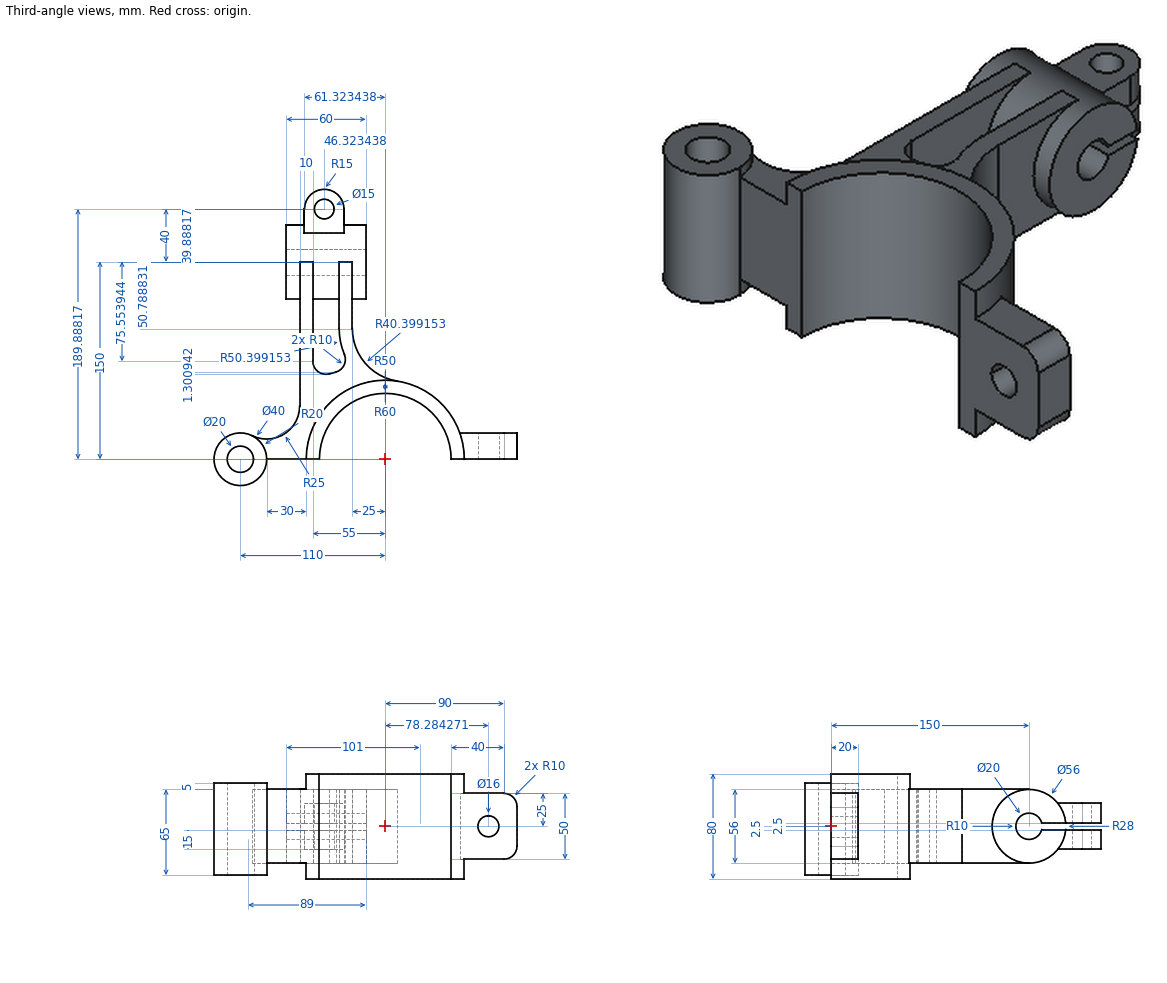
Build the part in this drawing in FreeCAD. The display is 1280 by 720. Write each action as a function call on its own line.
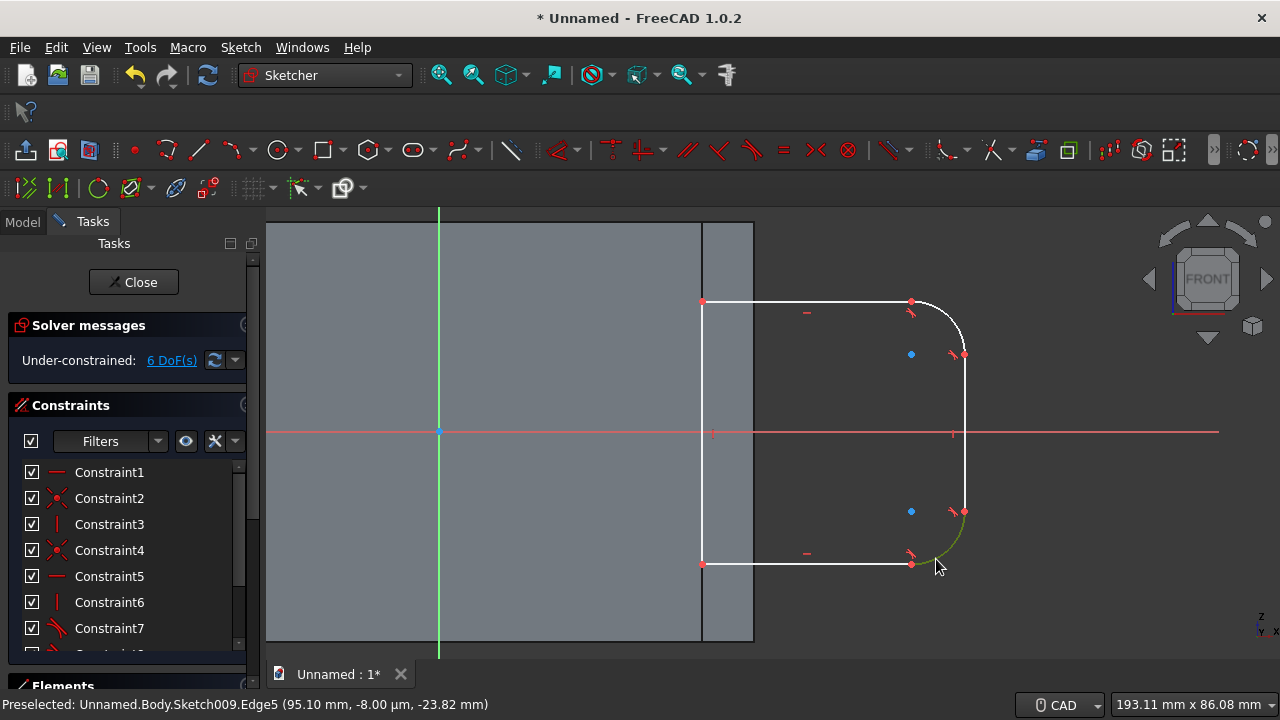
click(959, 330)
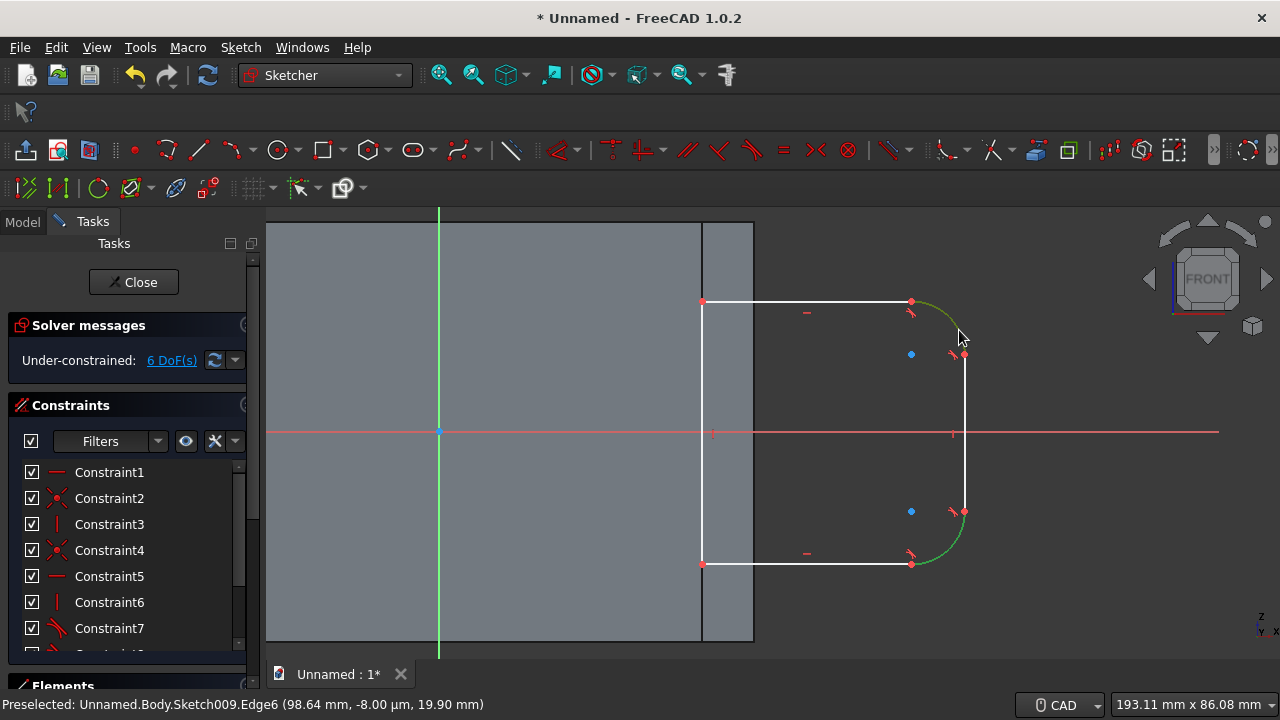
key(e)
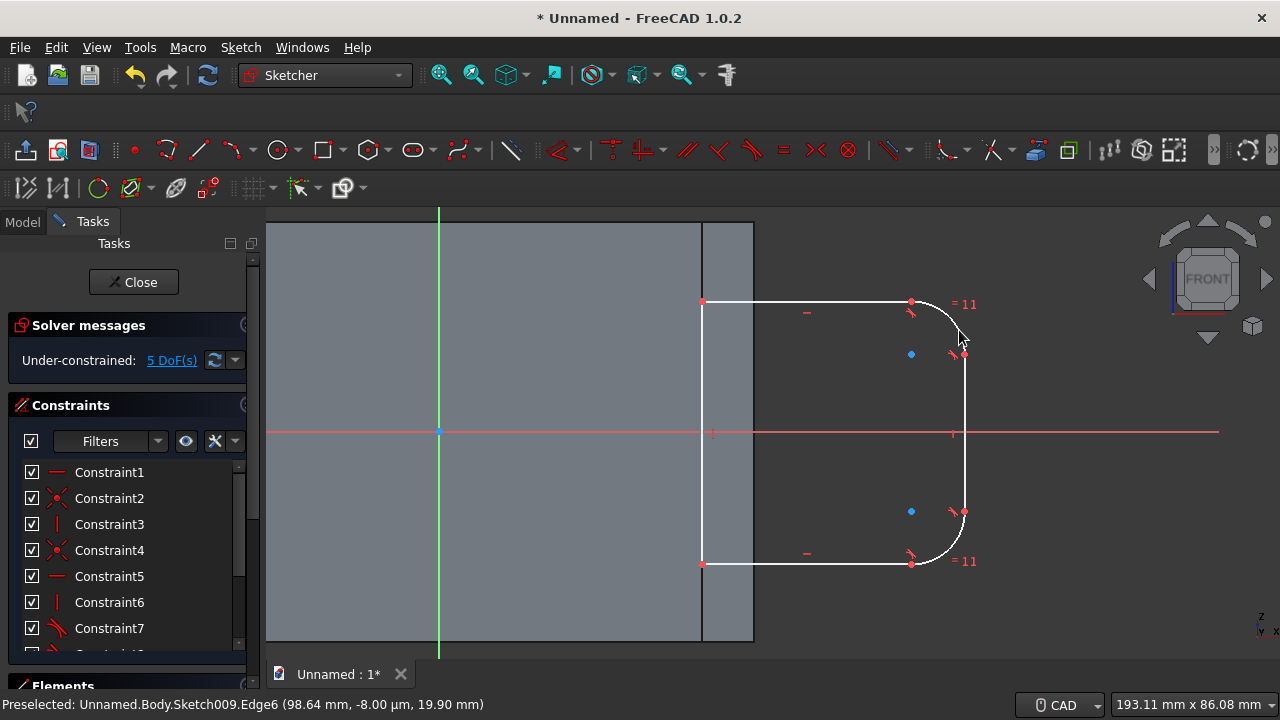
key(d)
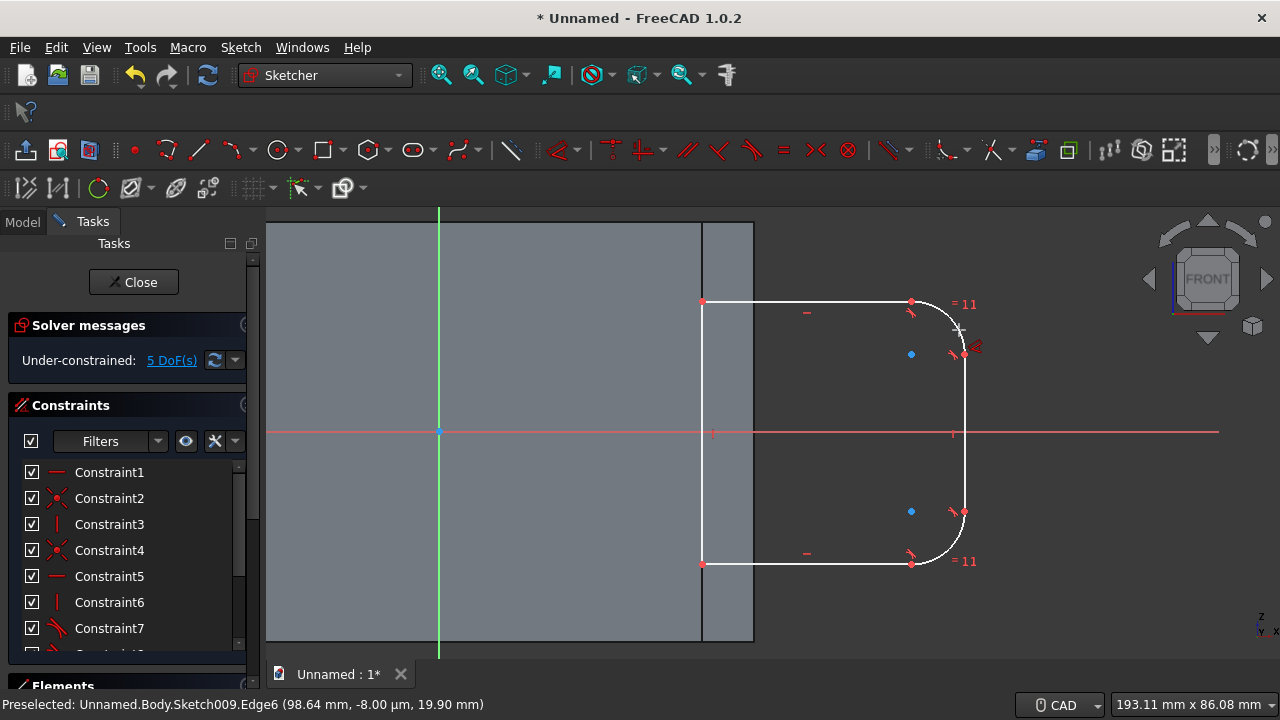
click(936, 559)
click(950, 588)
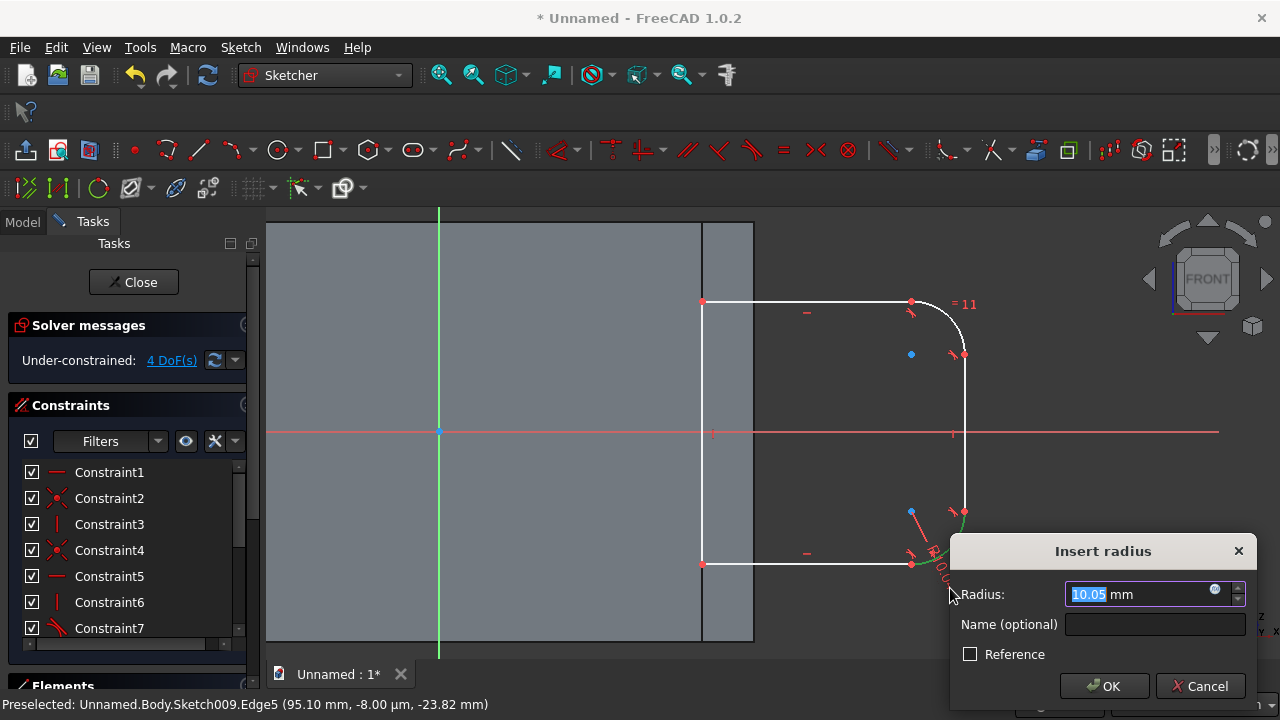
text(10)
key(Return)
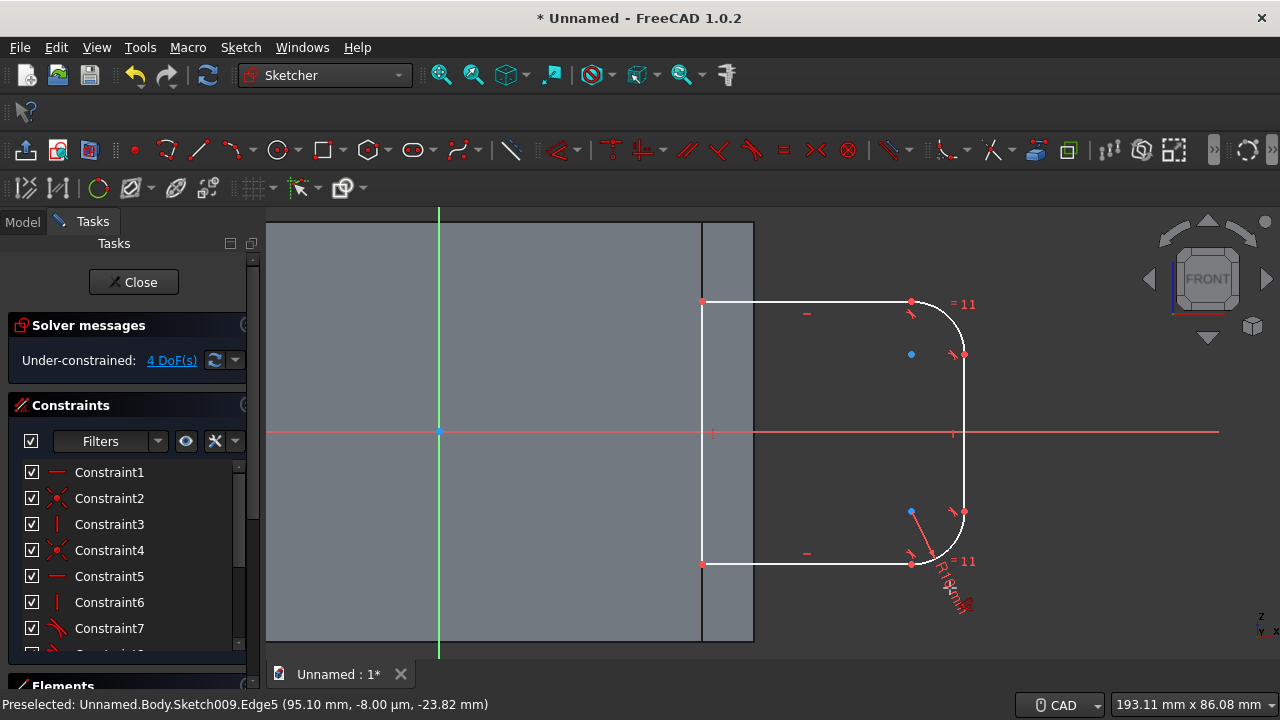
click(849, 302)
click(807, 268)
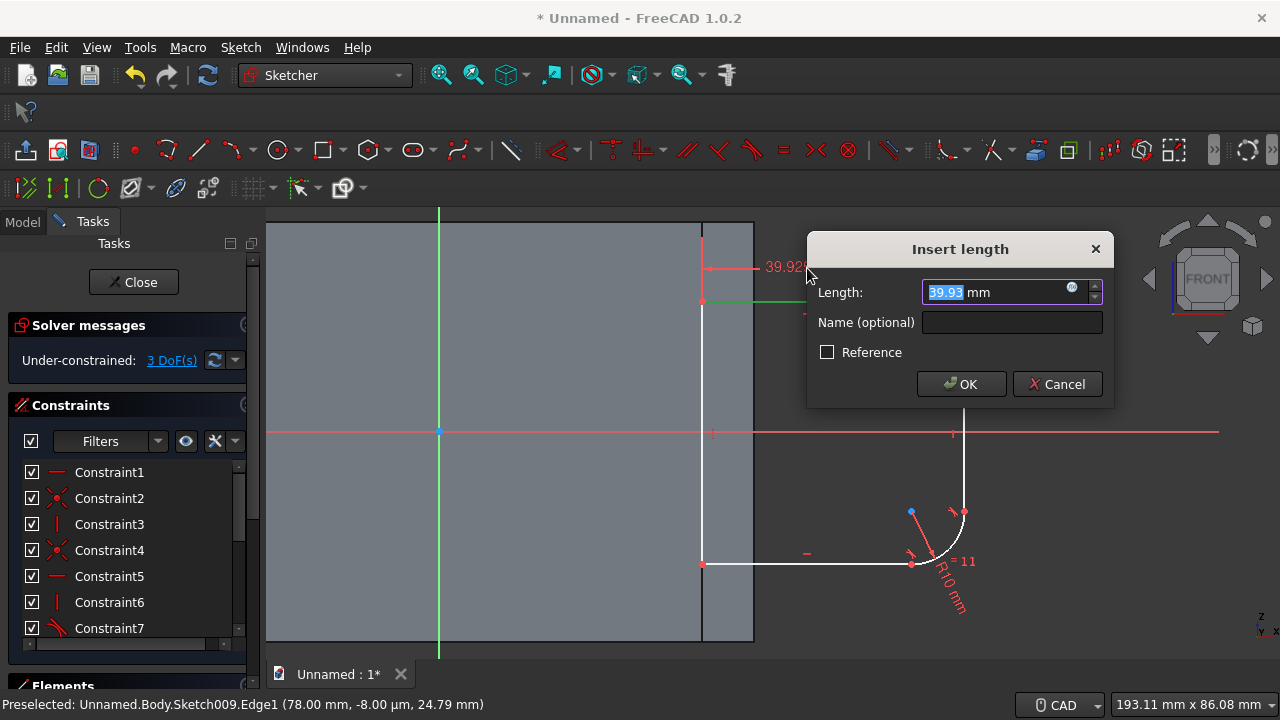
text(40)
key(Return)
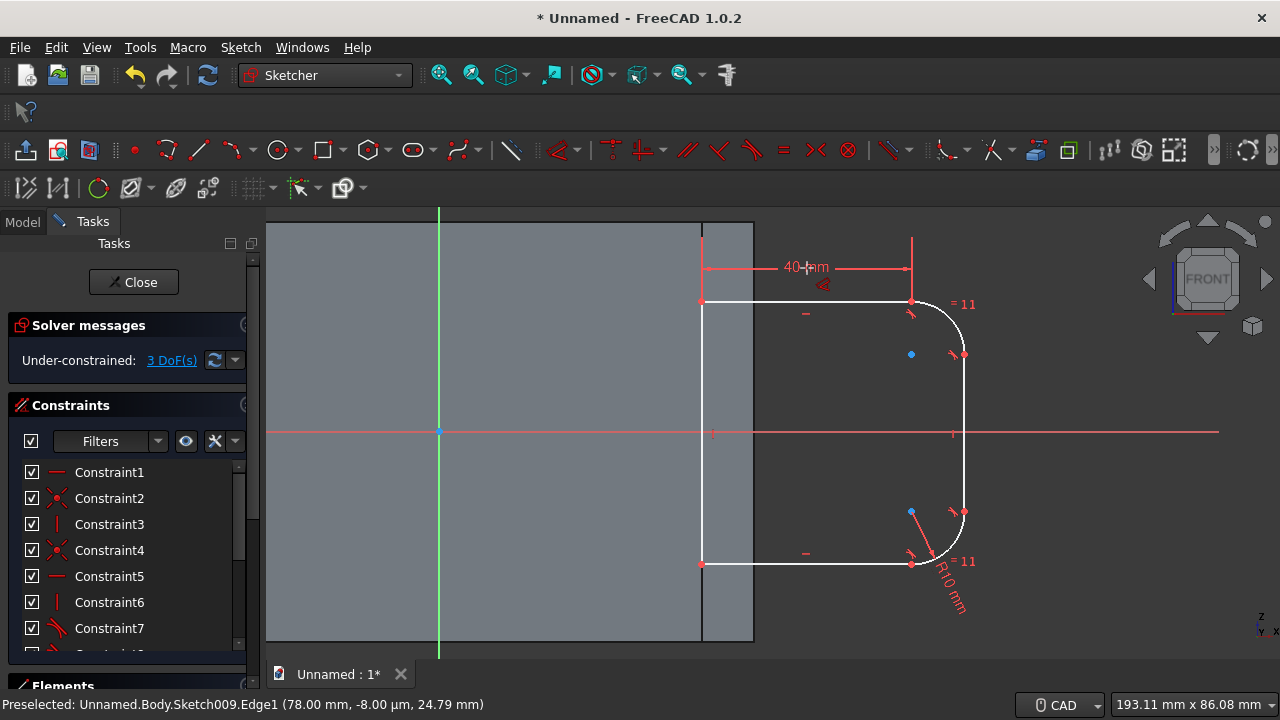
click(702, 381)
click(668, 373)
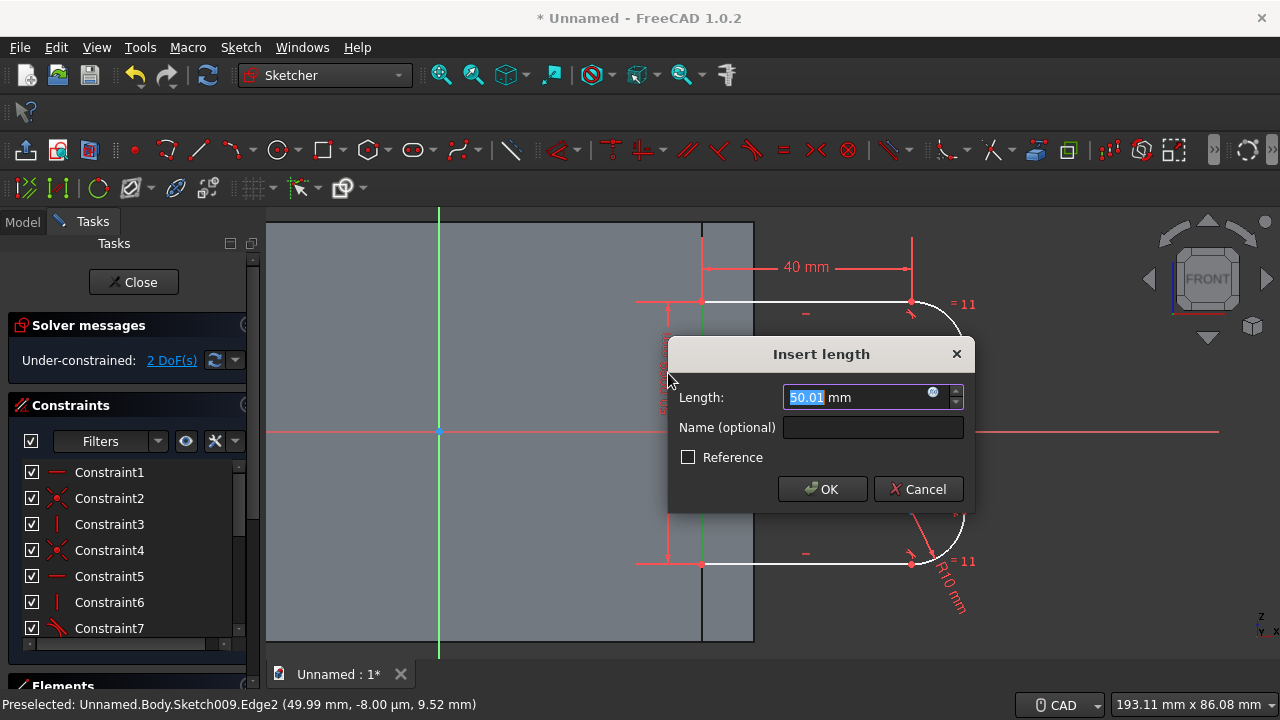
text(50)
key(Return)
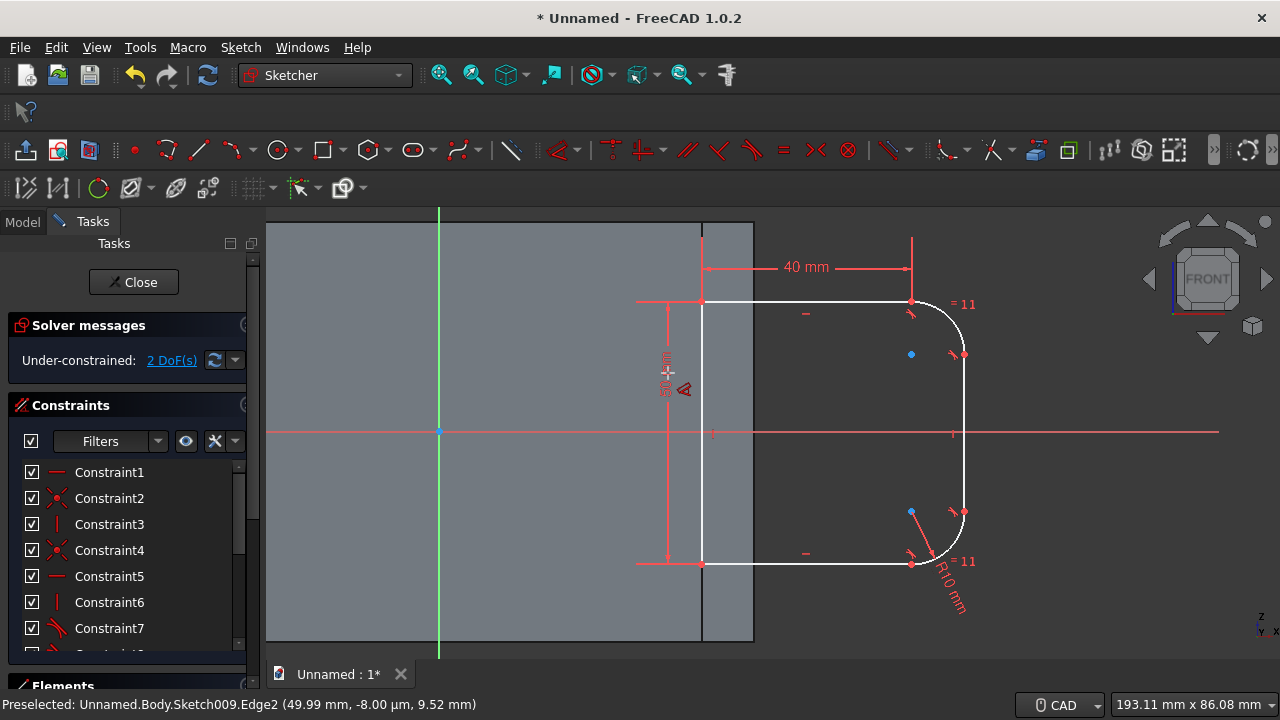
click(912, 302)
click(676, 268)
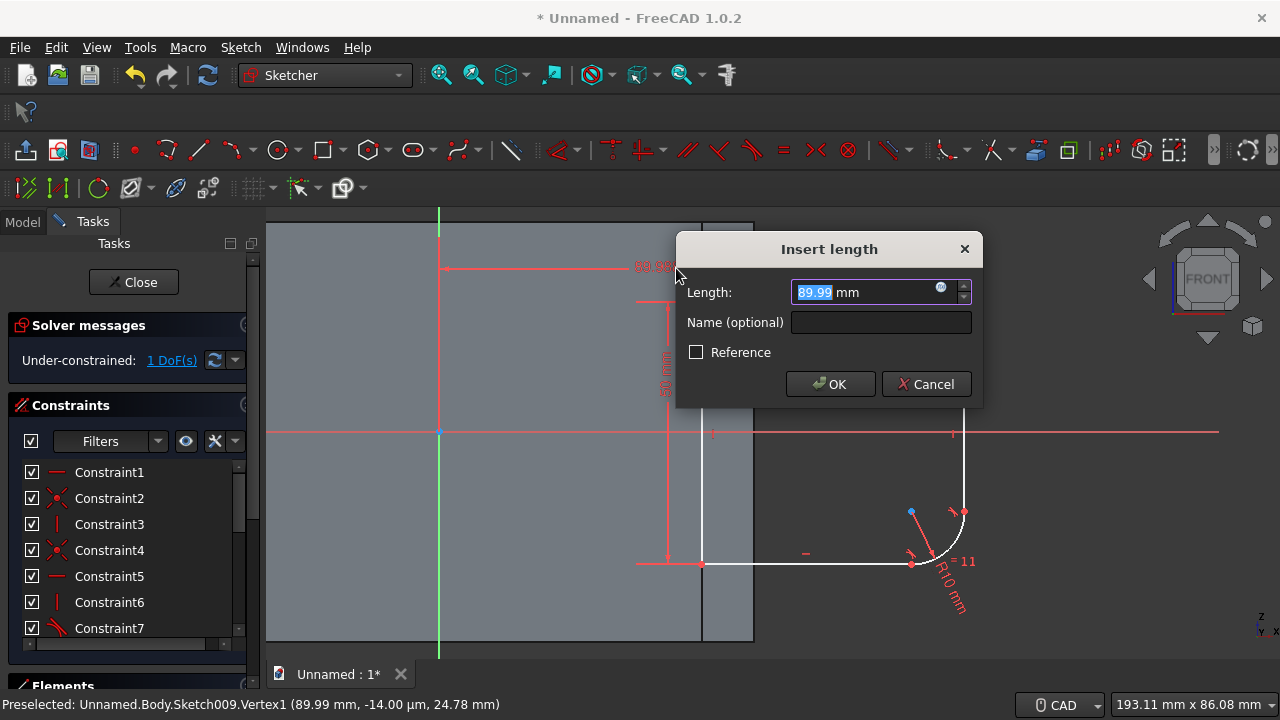
text(90)
key(Return)